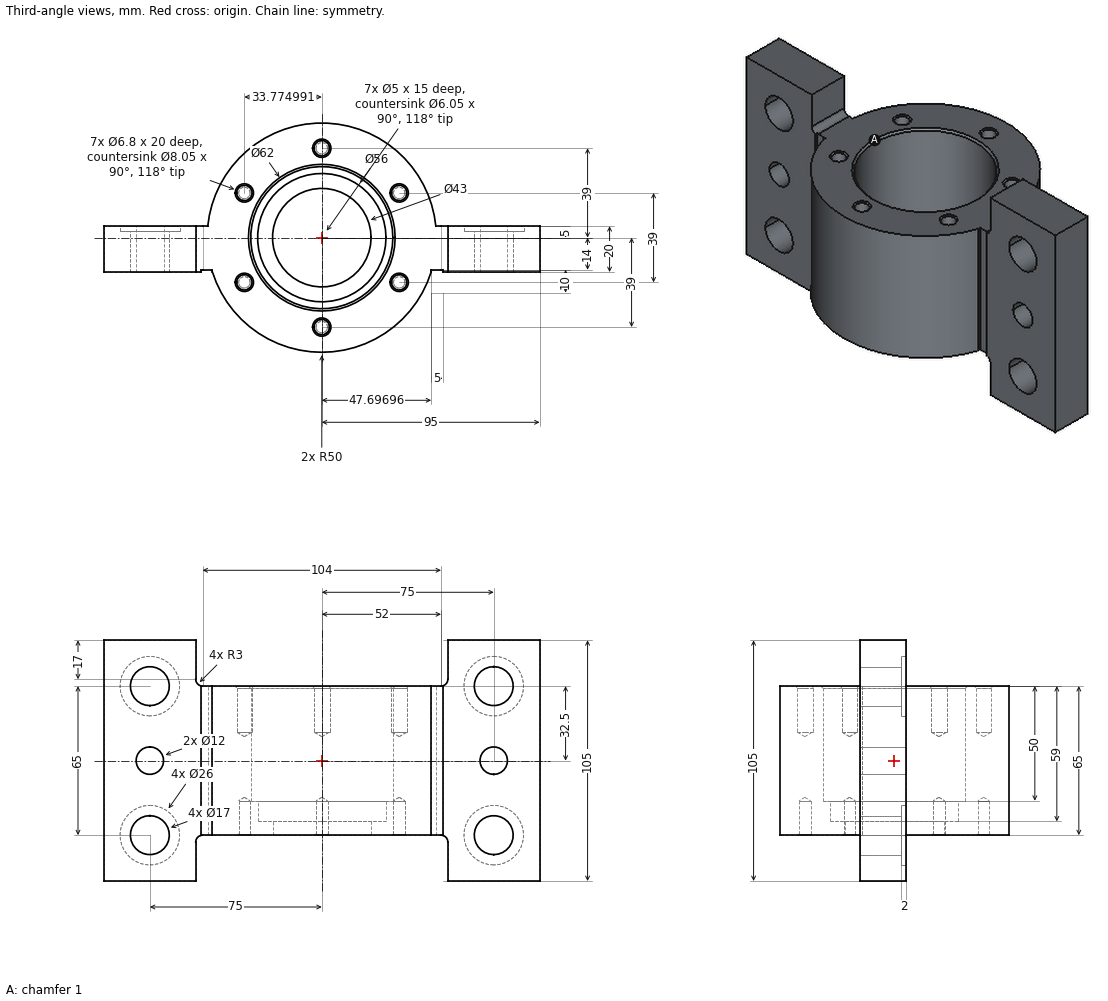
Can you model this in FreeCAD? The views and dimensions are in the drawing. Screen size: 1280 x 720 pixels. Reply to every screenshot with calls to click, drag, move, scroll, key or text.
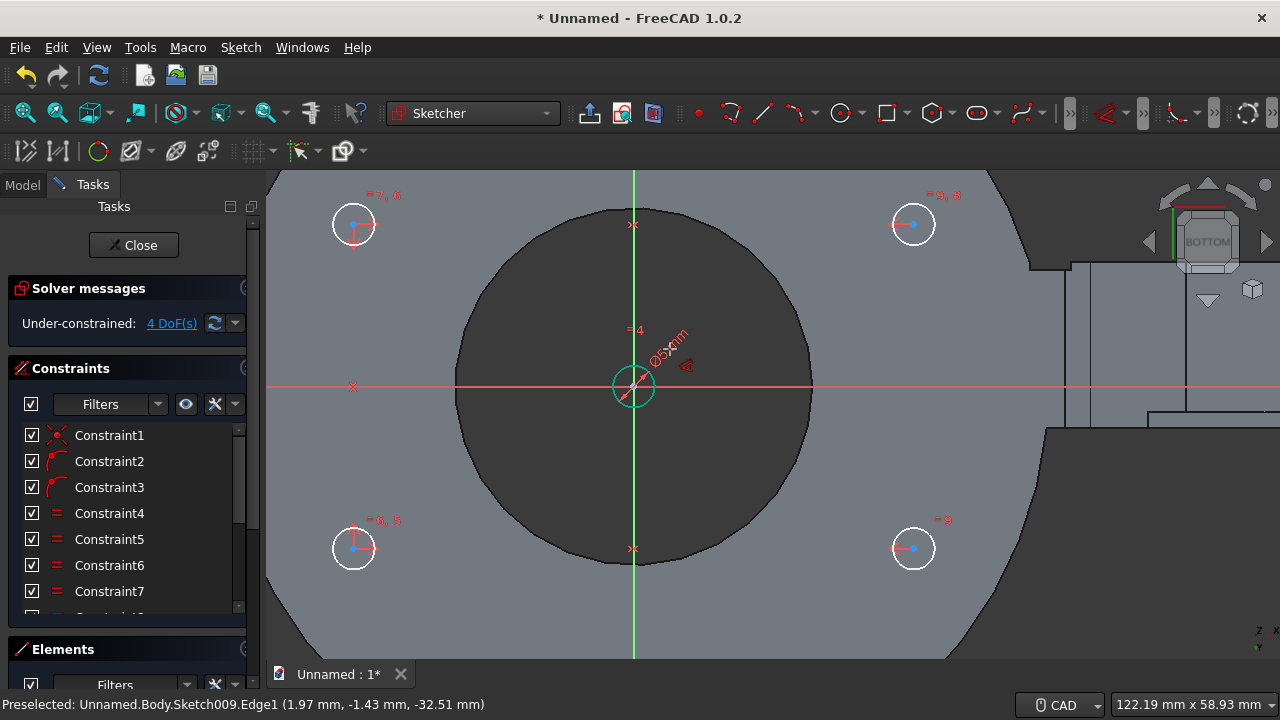
scroll(762, 437, down, 4)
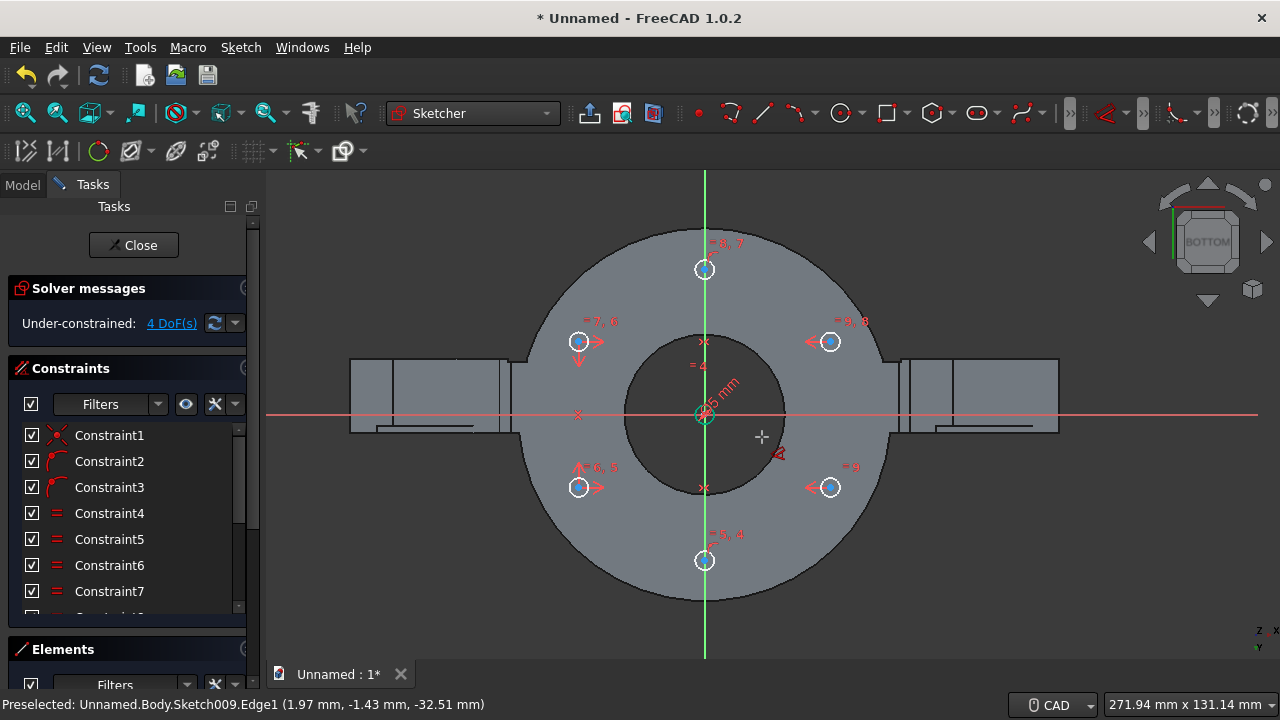
click(705, 561)
click(739, 488)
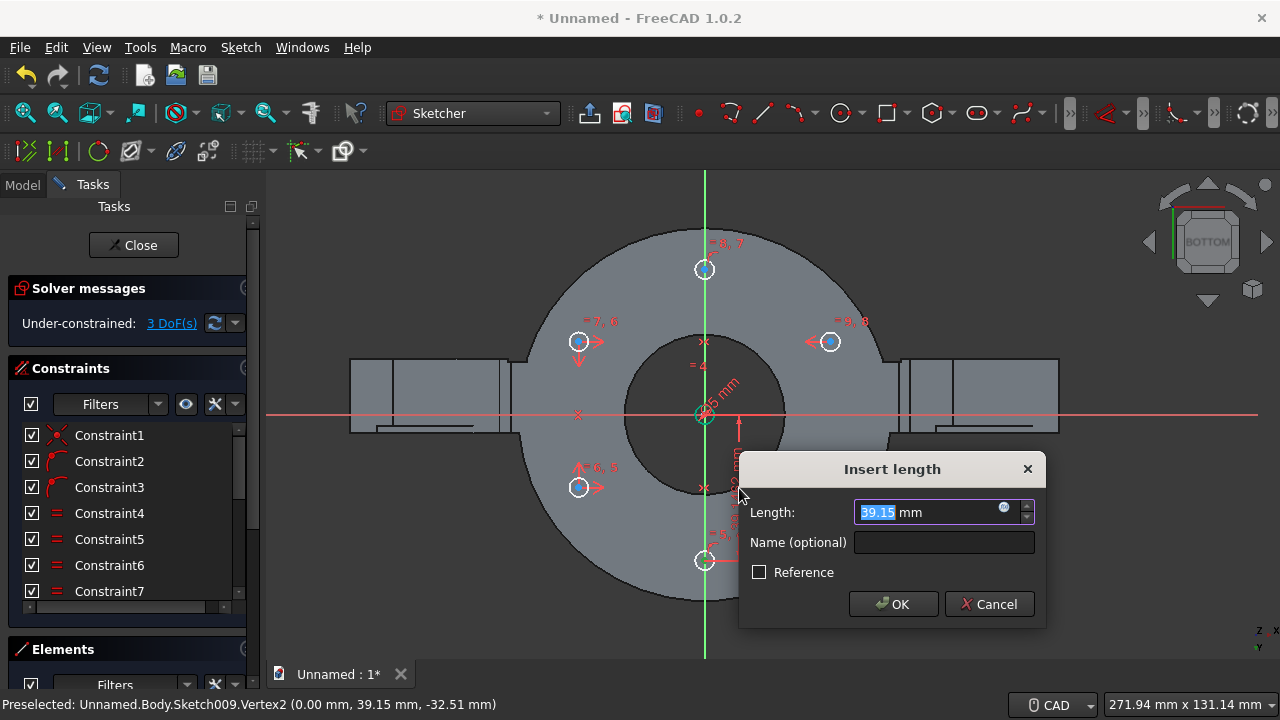
text(39)
key(Return)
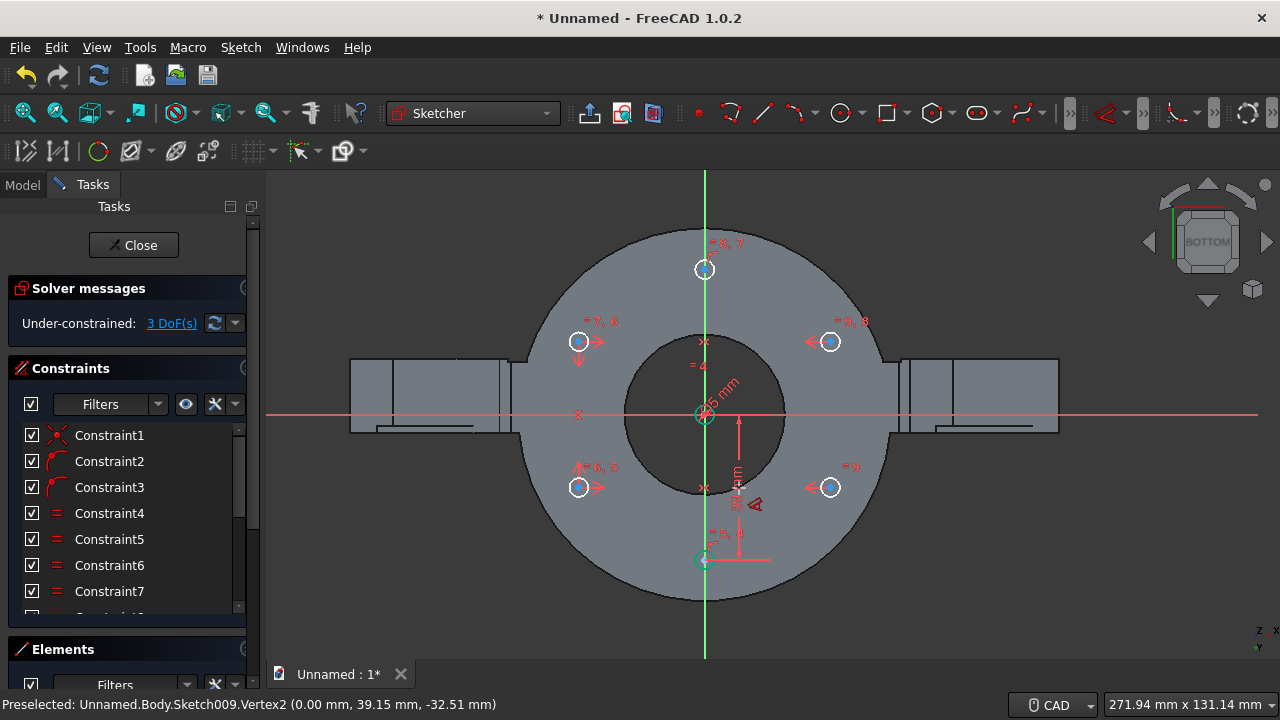
click(705, 270)
click(739, 342)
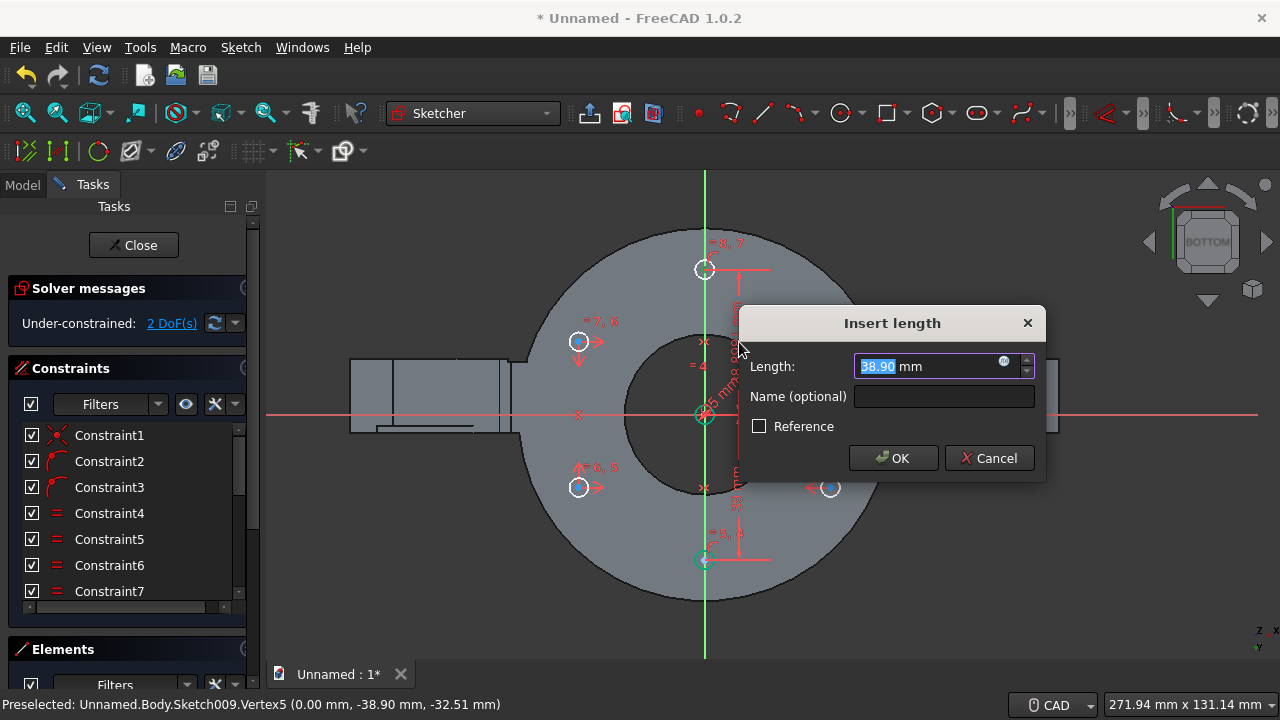
text(39)
key(Return)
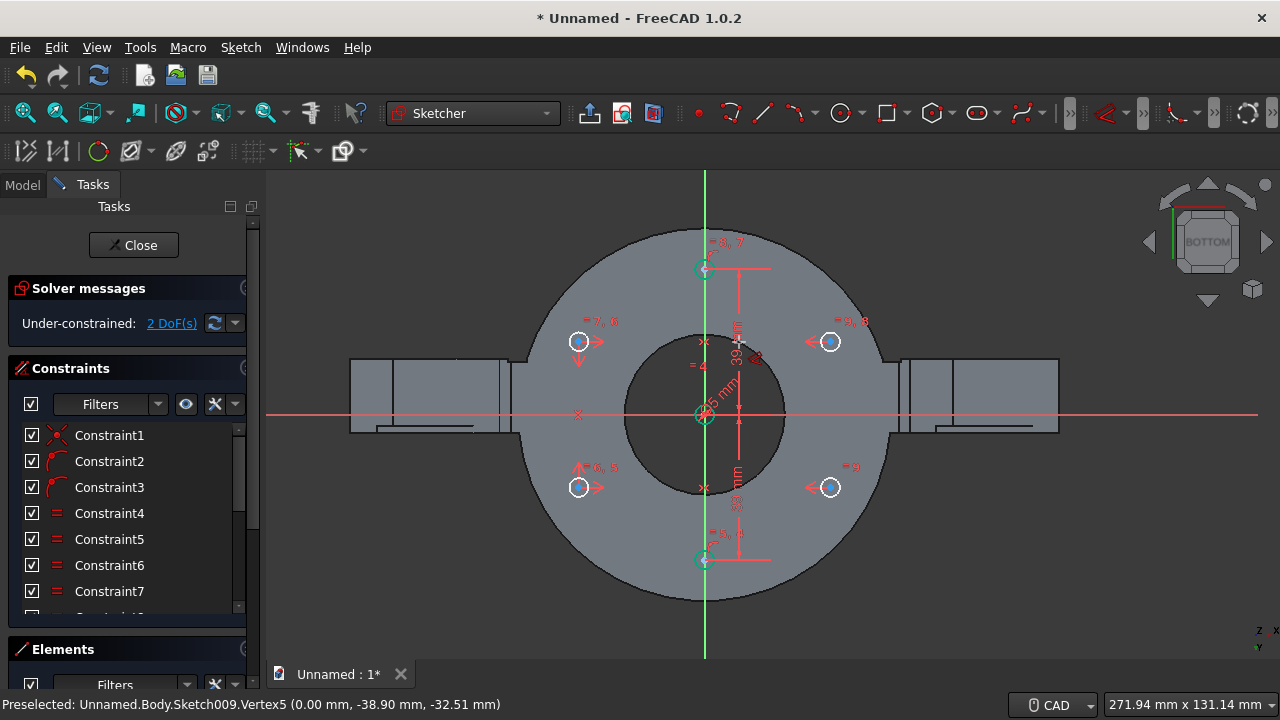
click(579, 488)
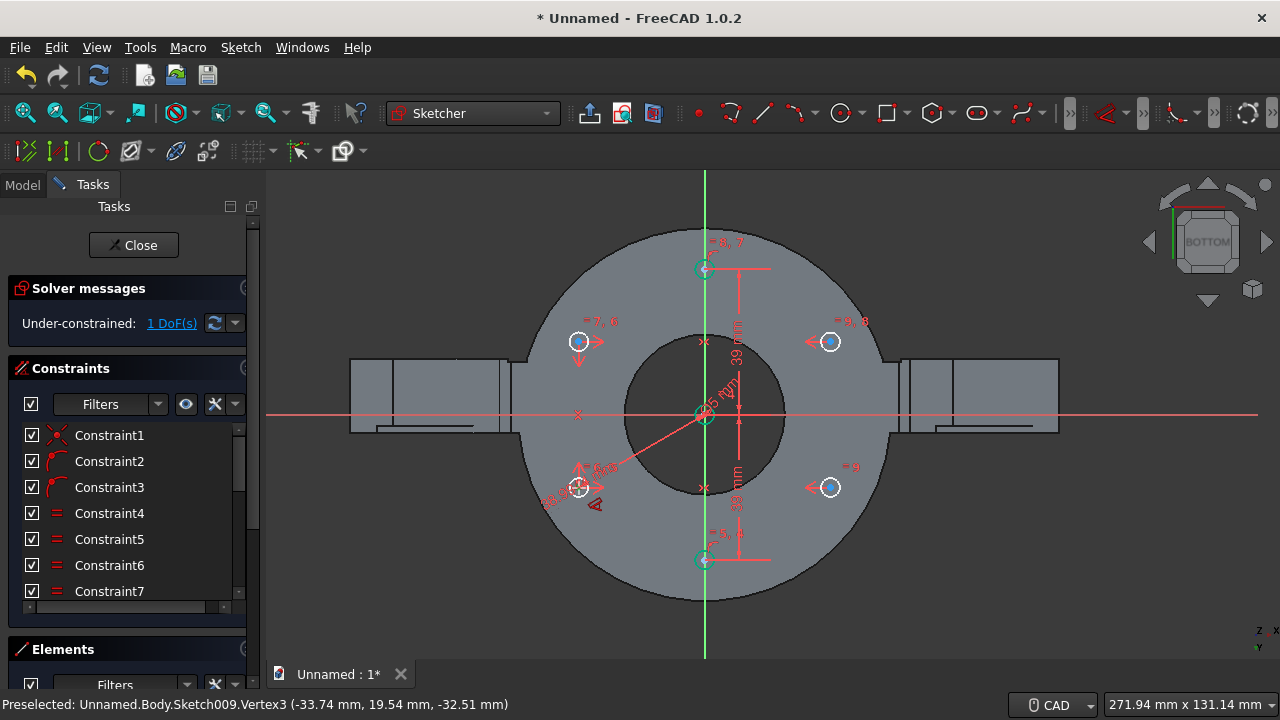
click(579, 342)
click(545, 381)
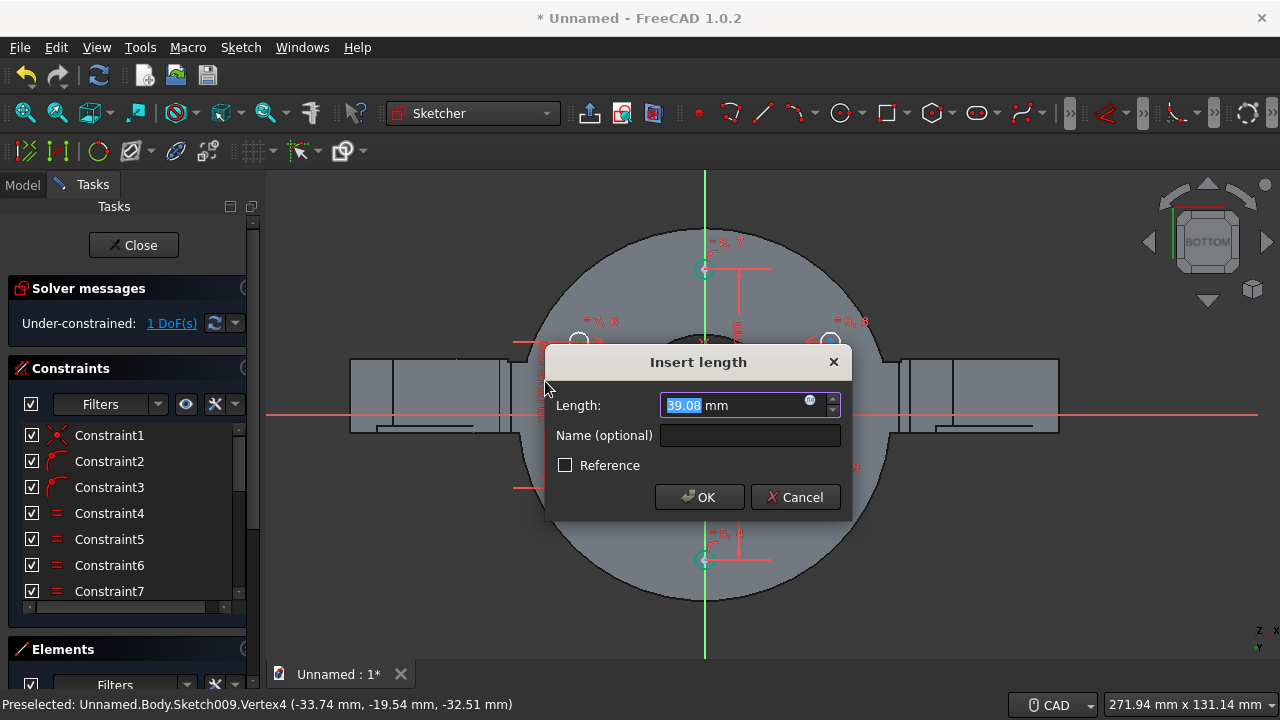
text(39)
key(Return)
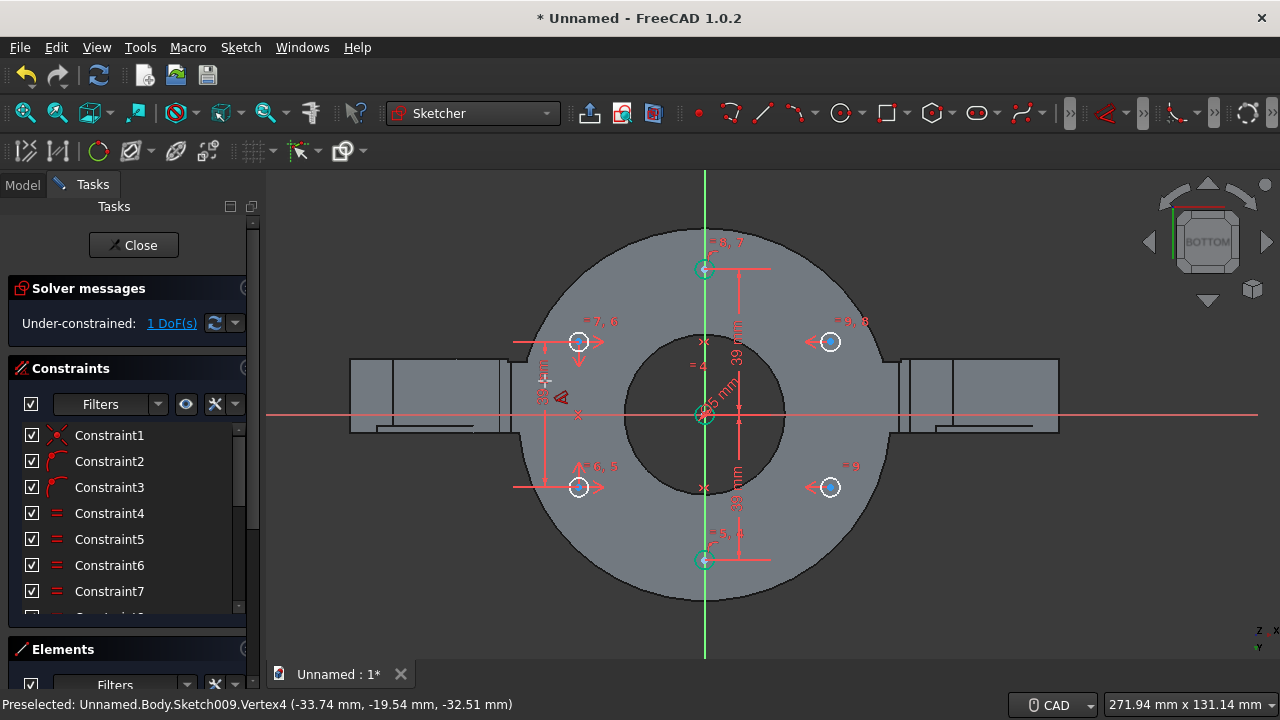
click(579, 487)
click(642, 521)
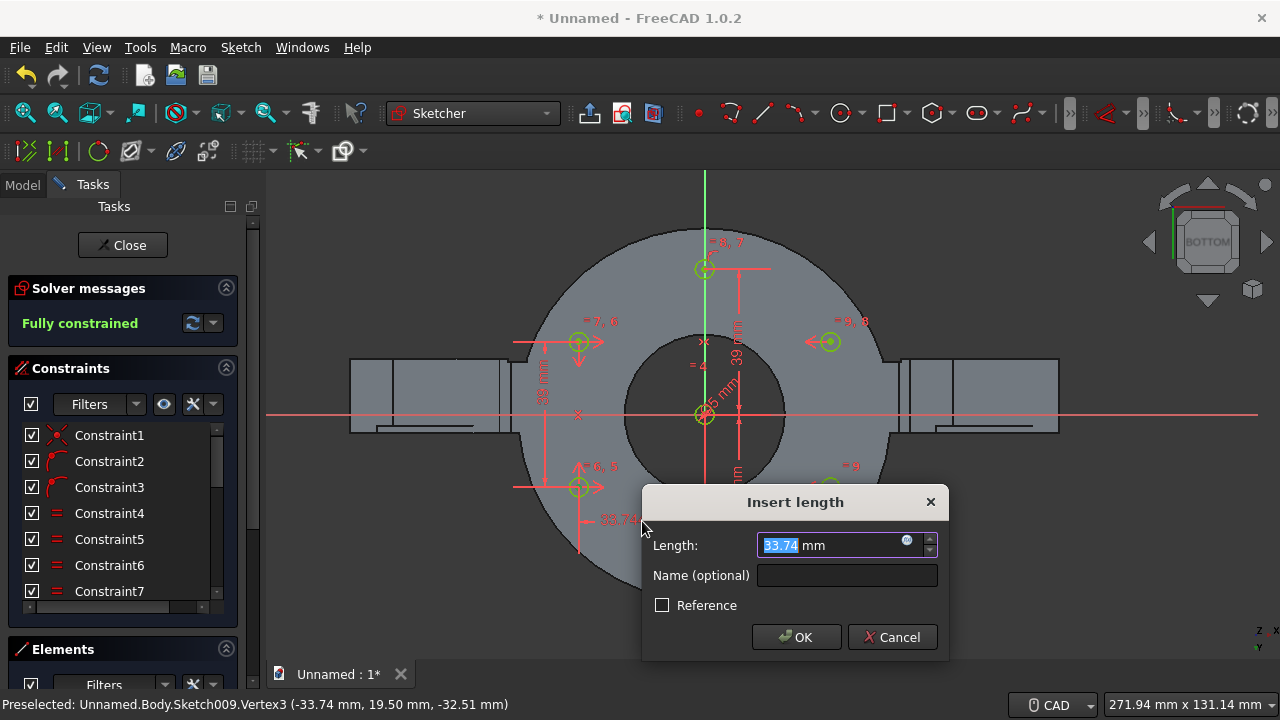
text(33.774991)
key(Return)
key(Escape)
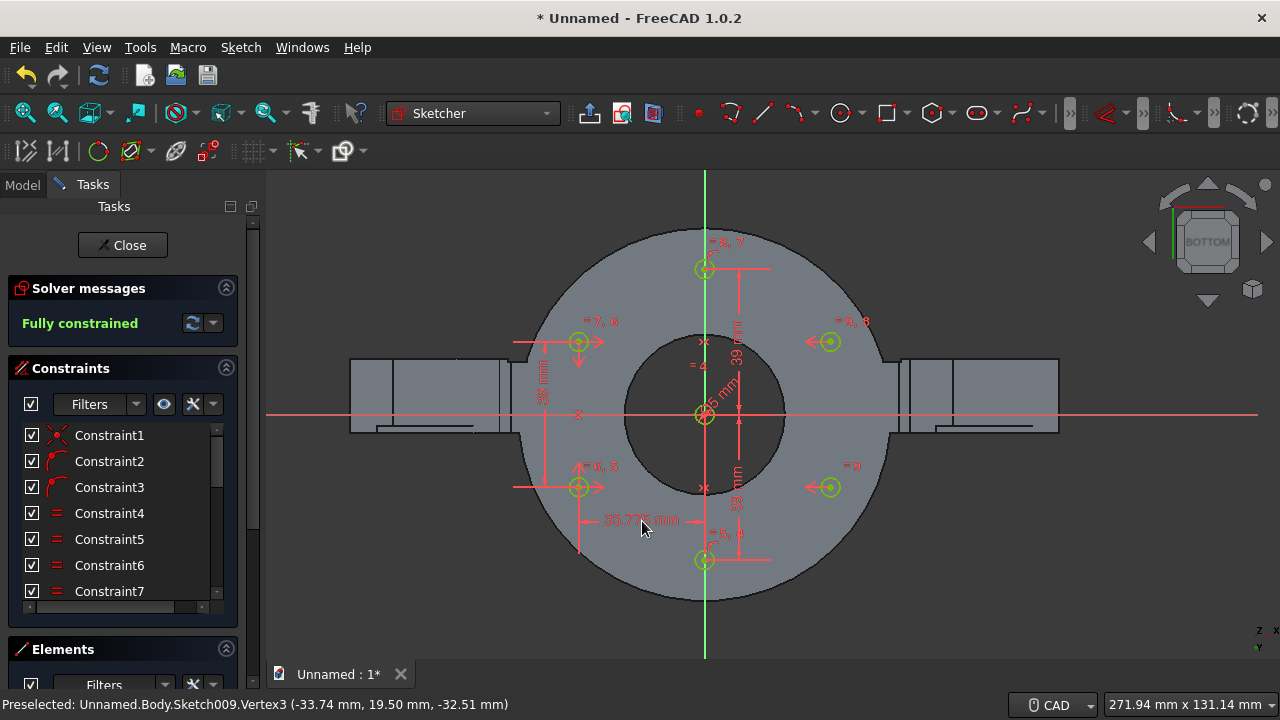
click(123, 245)